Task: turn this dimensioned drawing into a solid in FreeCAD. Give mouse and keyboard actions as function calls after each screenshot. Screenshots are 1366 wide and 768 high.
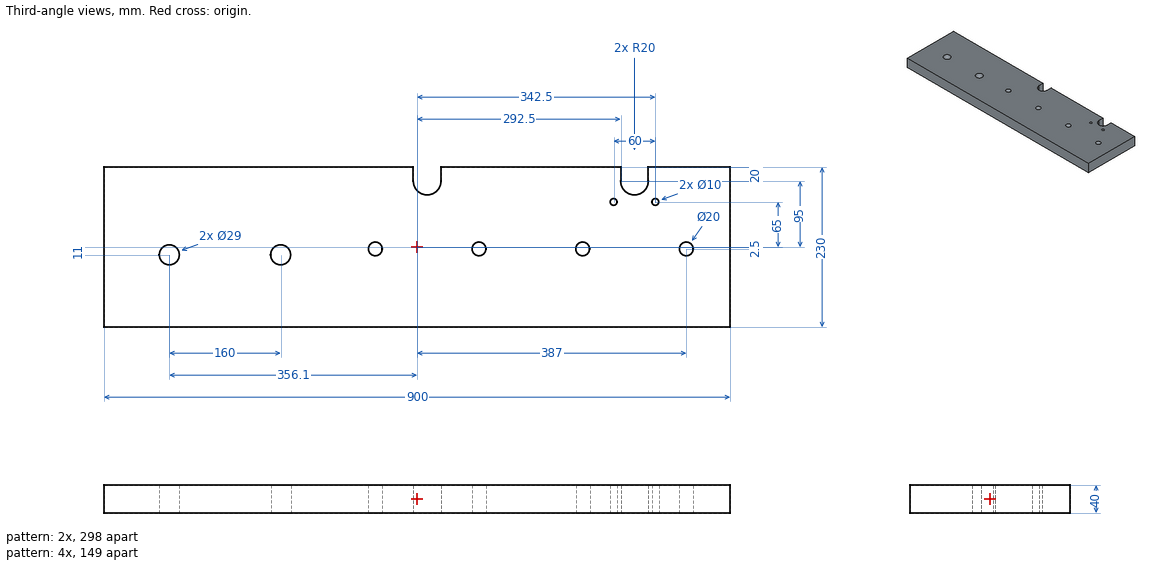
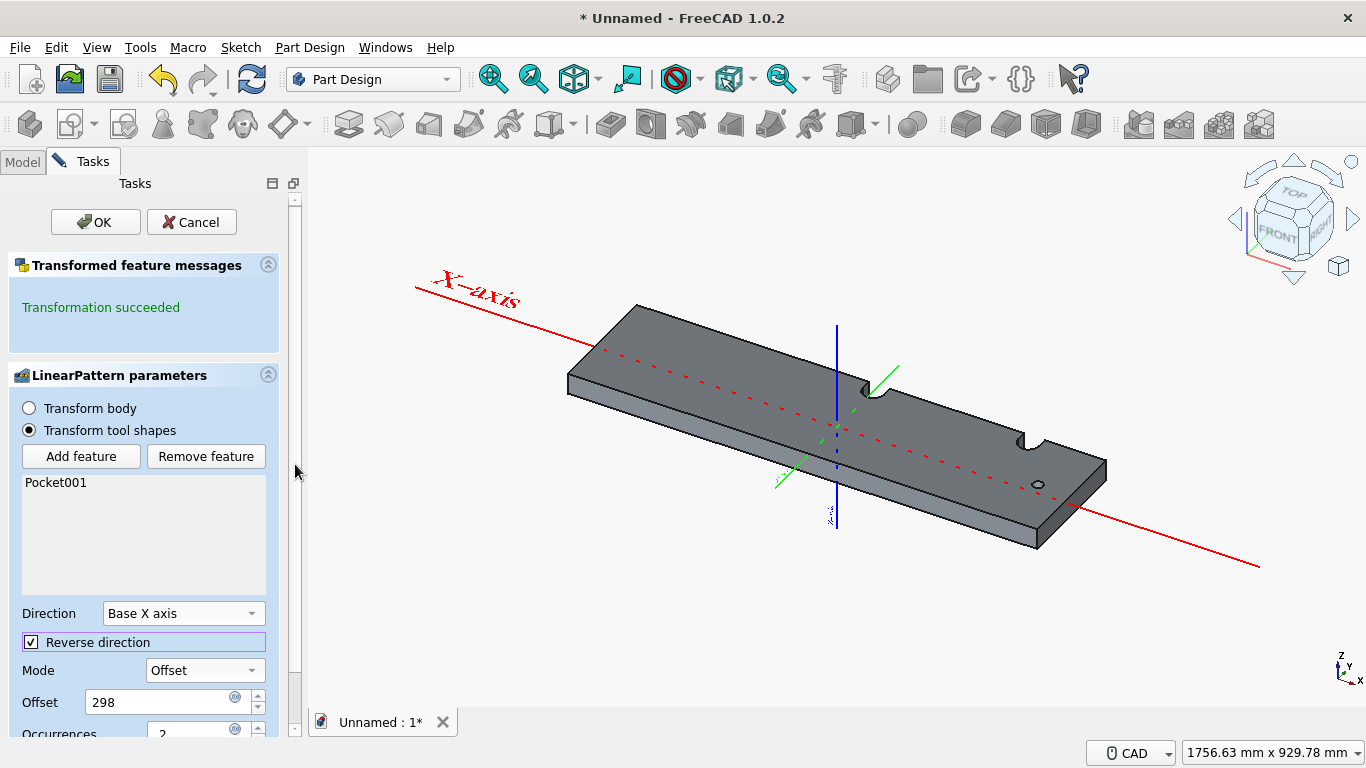
click(96, 222)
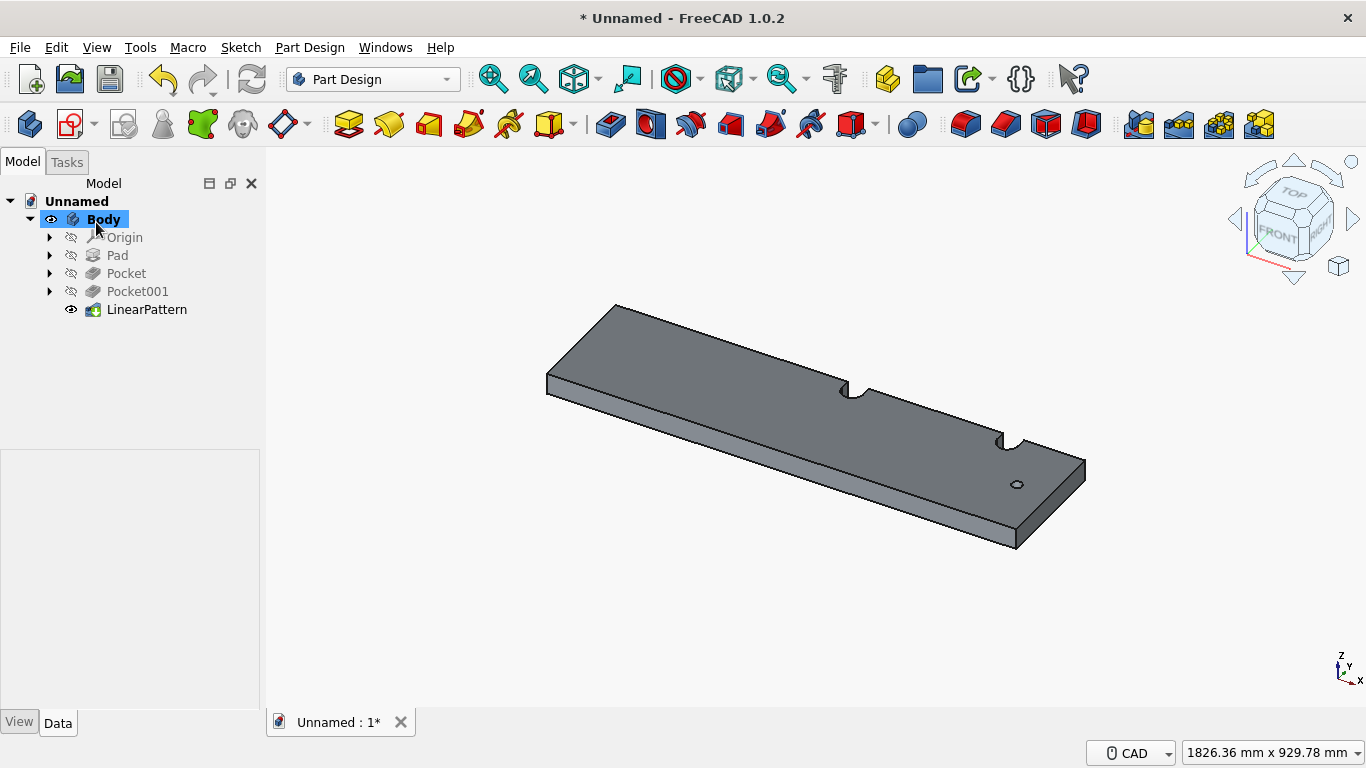
click(116, 273)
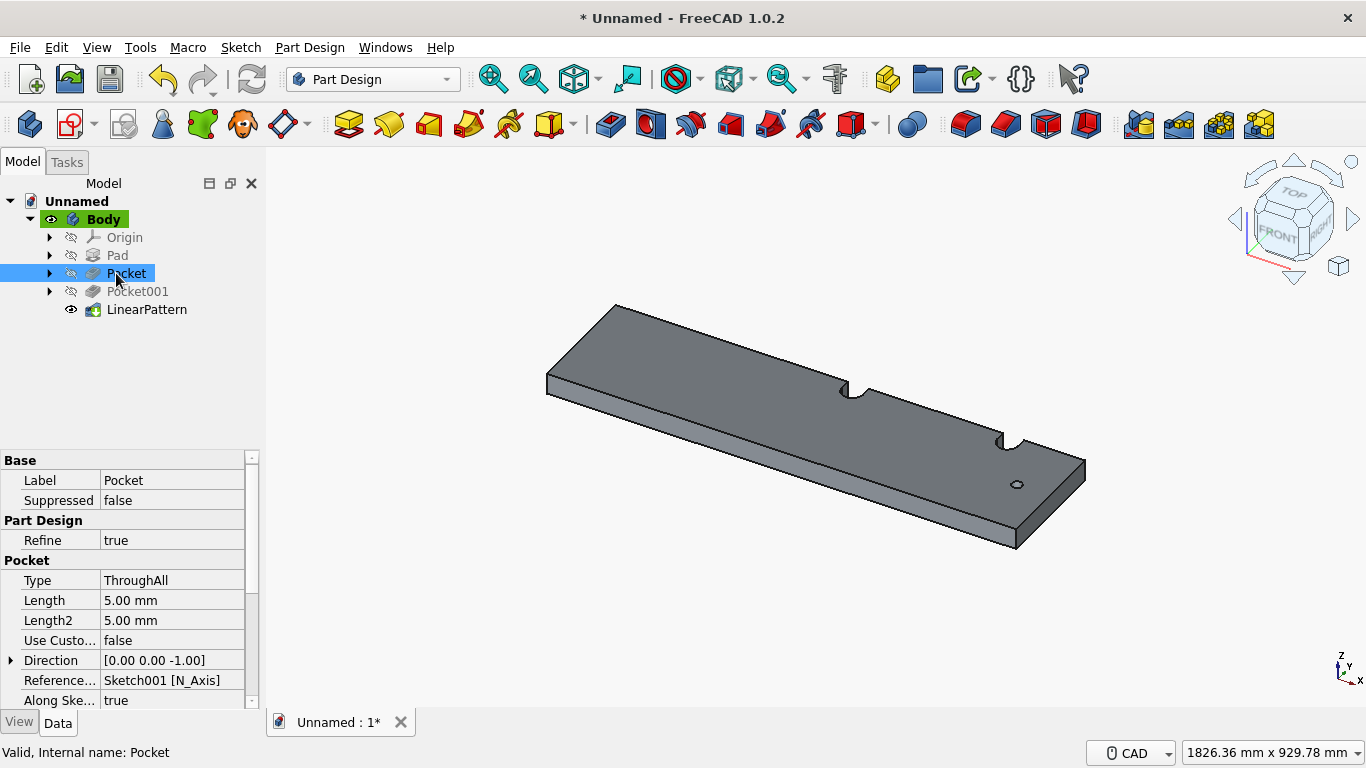
click(1180, 124)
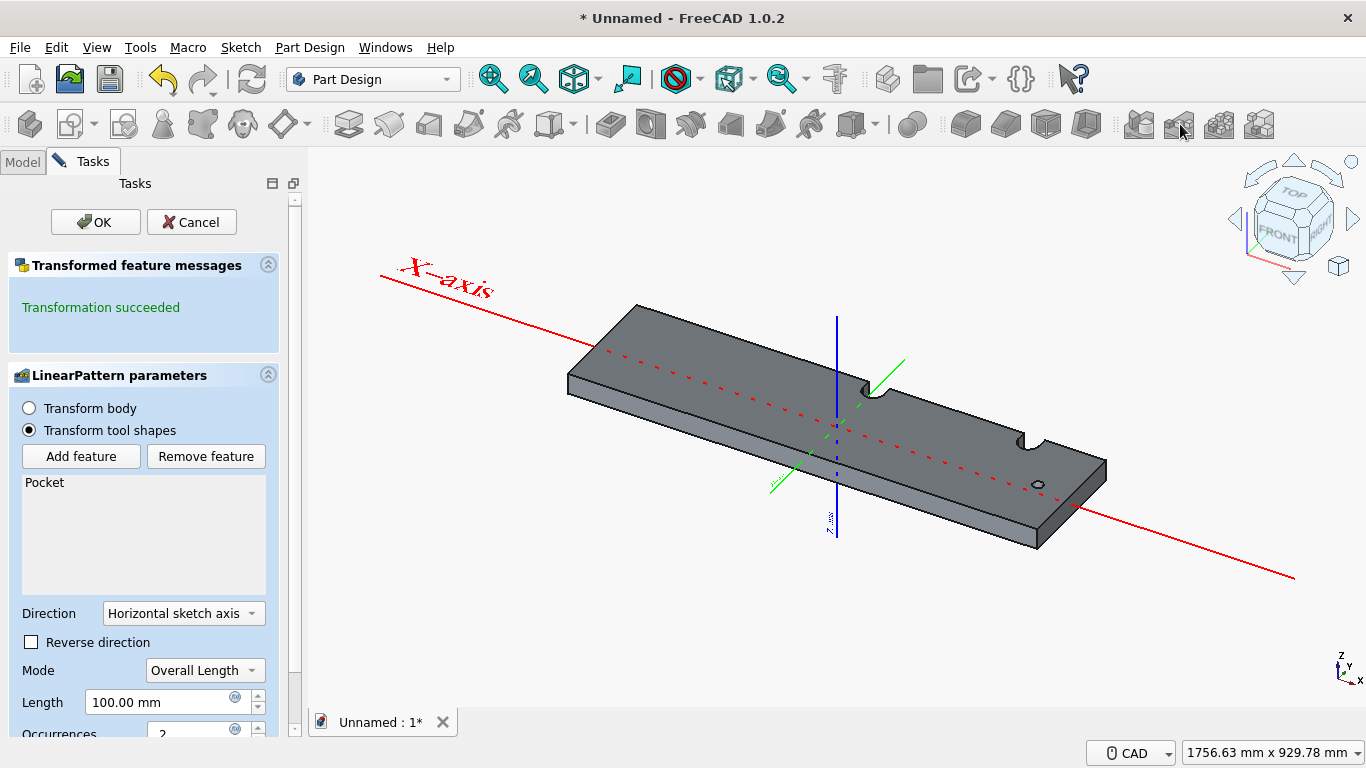
click(184, 614)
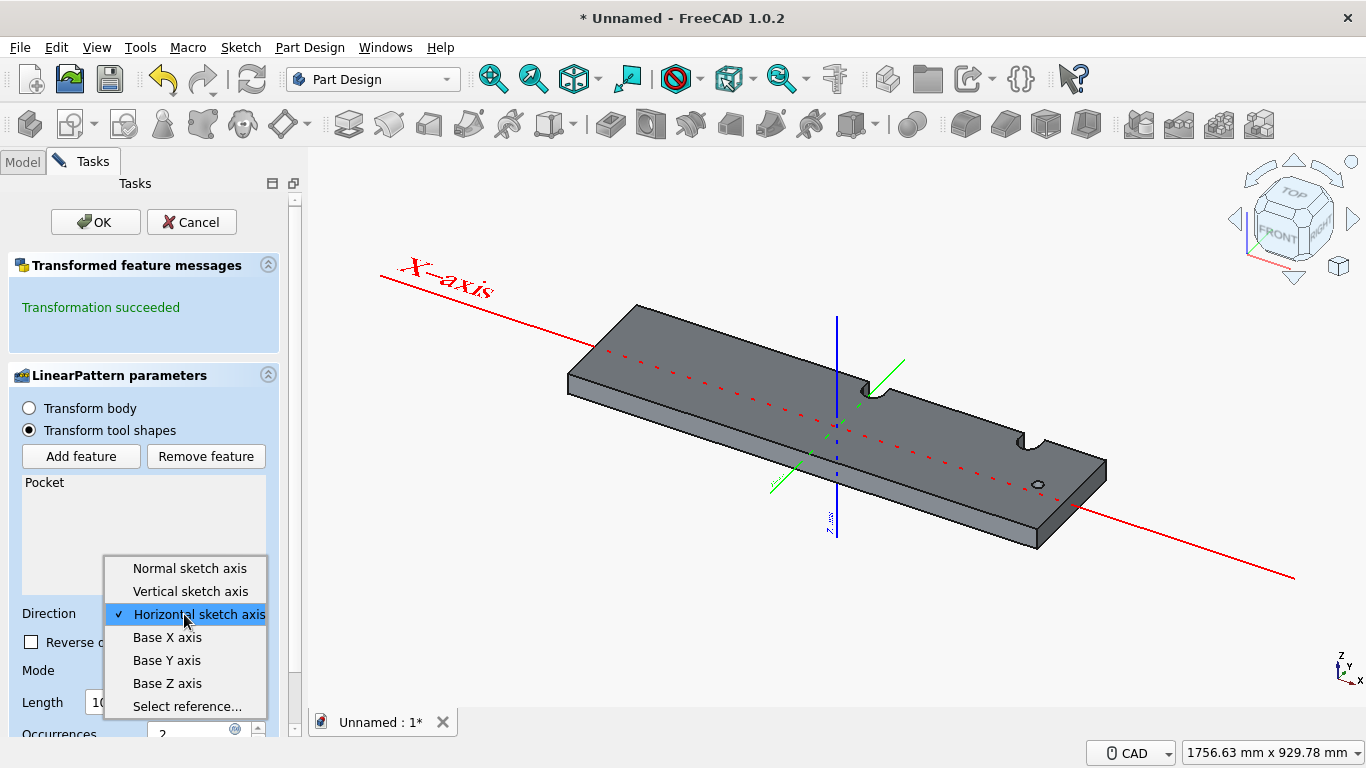
click(184, 638)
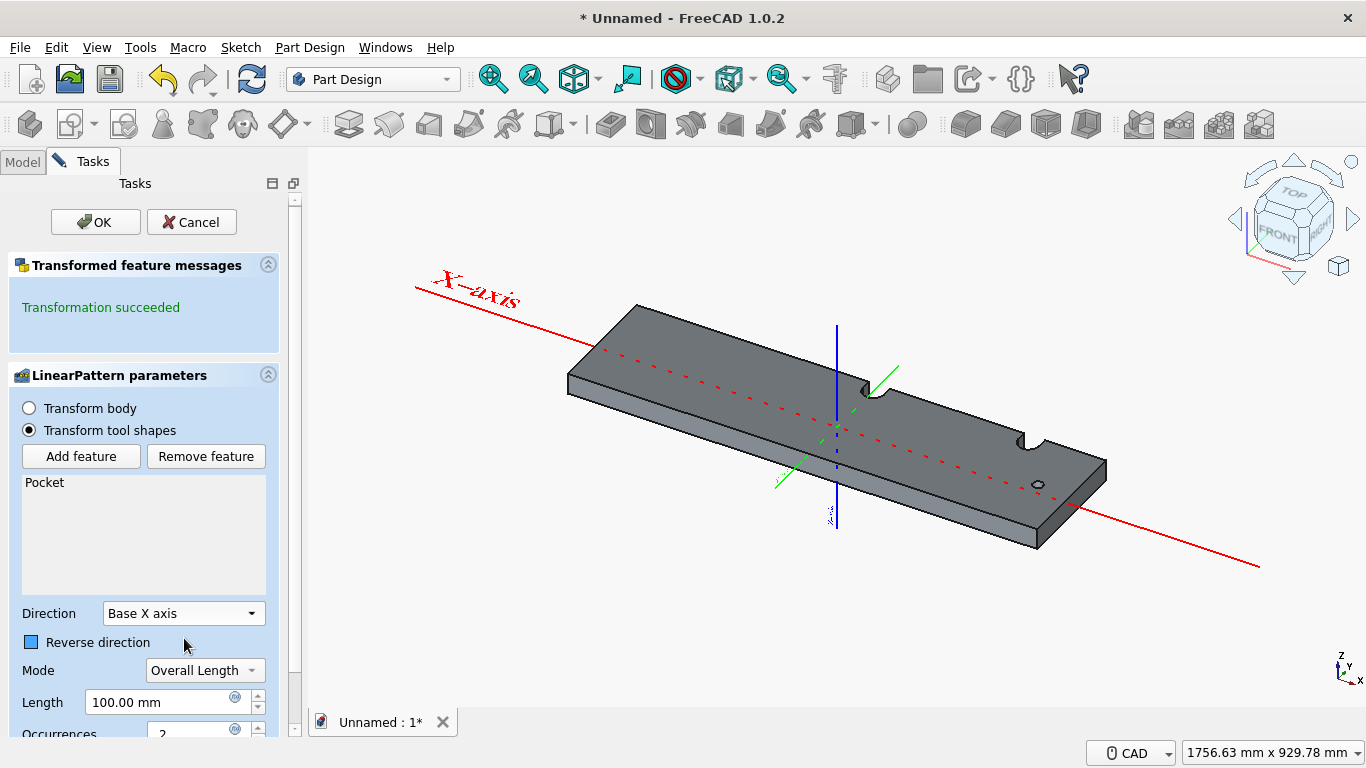
click(206, 670)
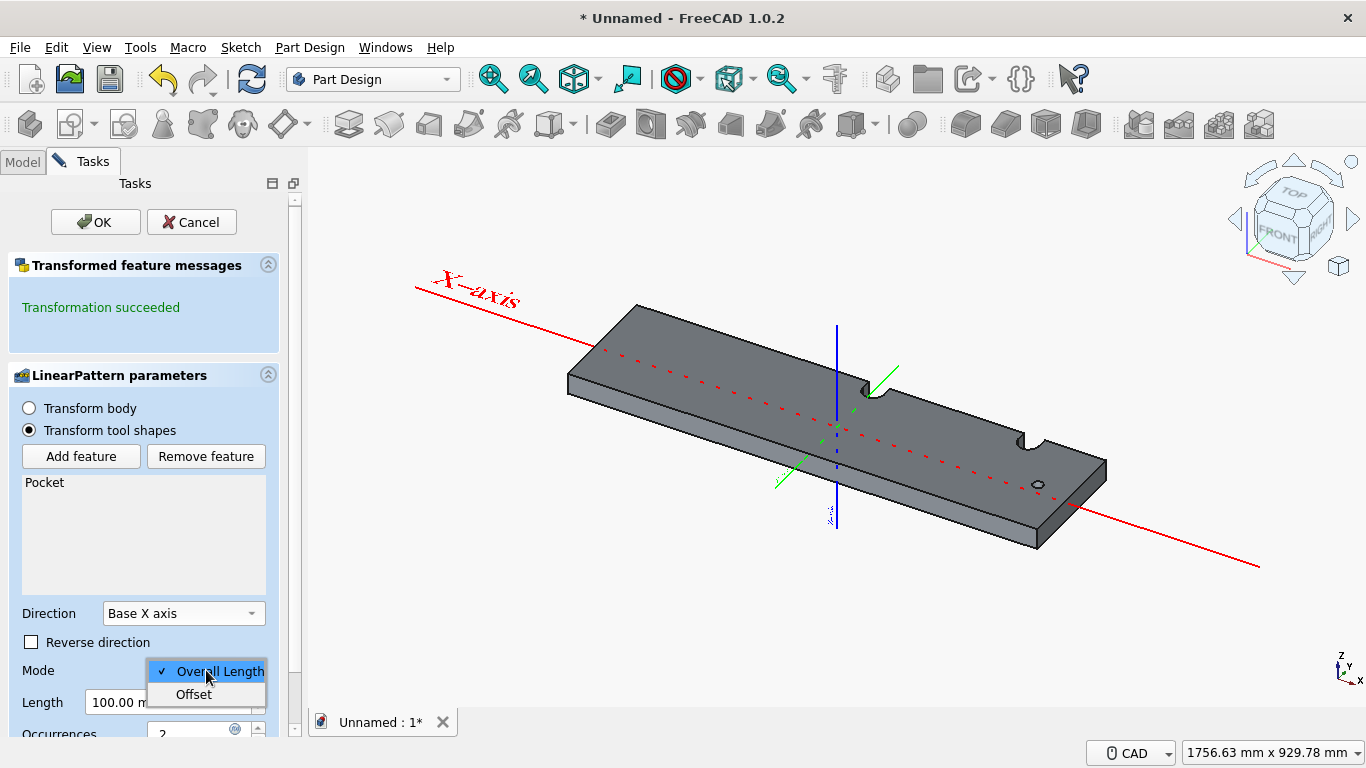
click(206, 694)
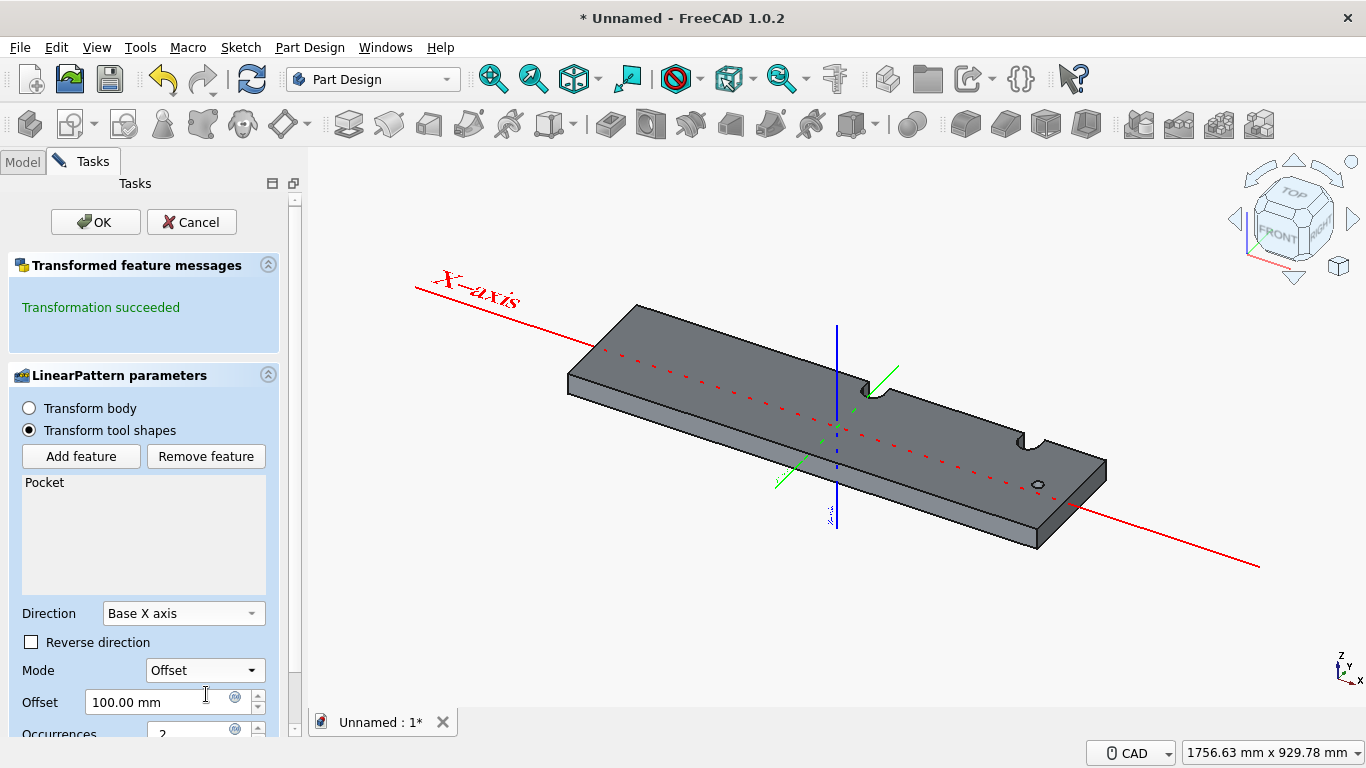
triple_click(168, 702)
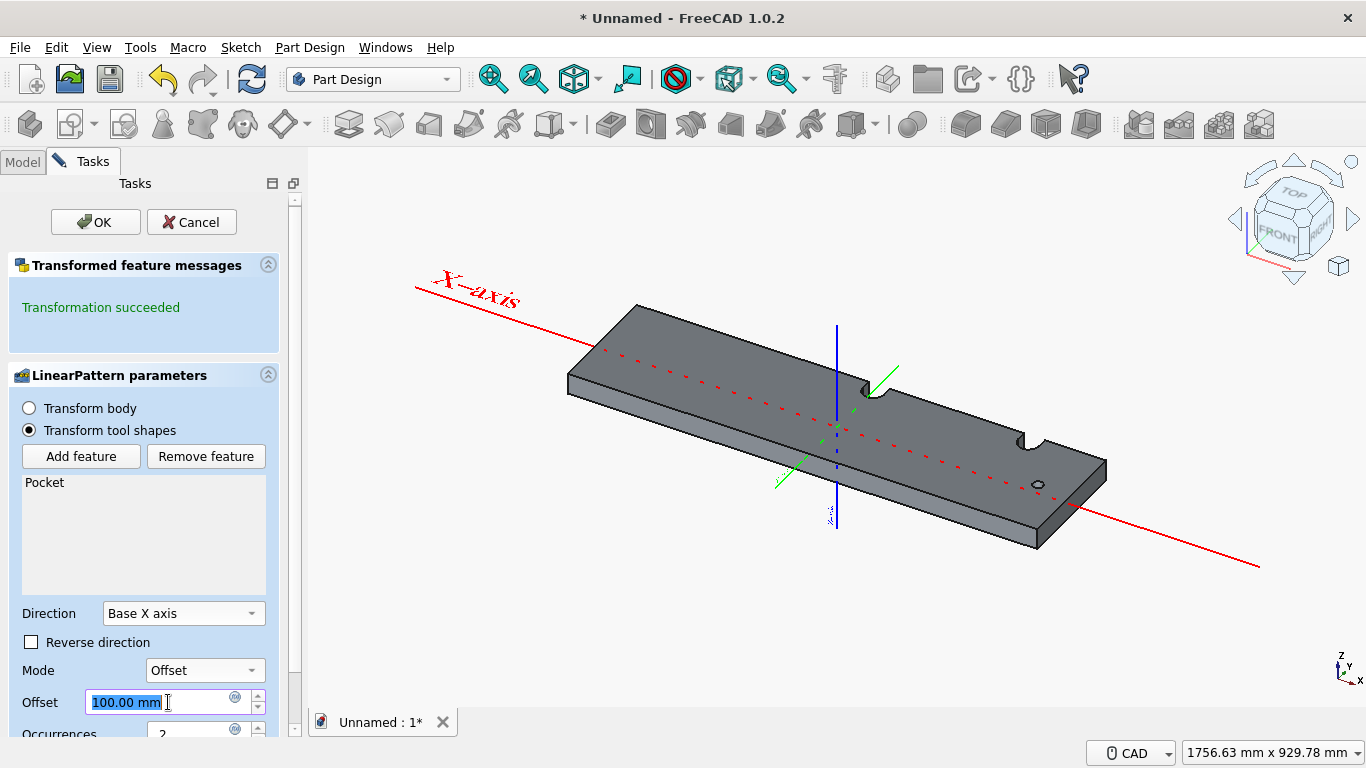
text(149)
key(Tab)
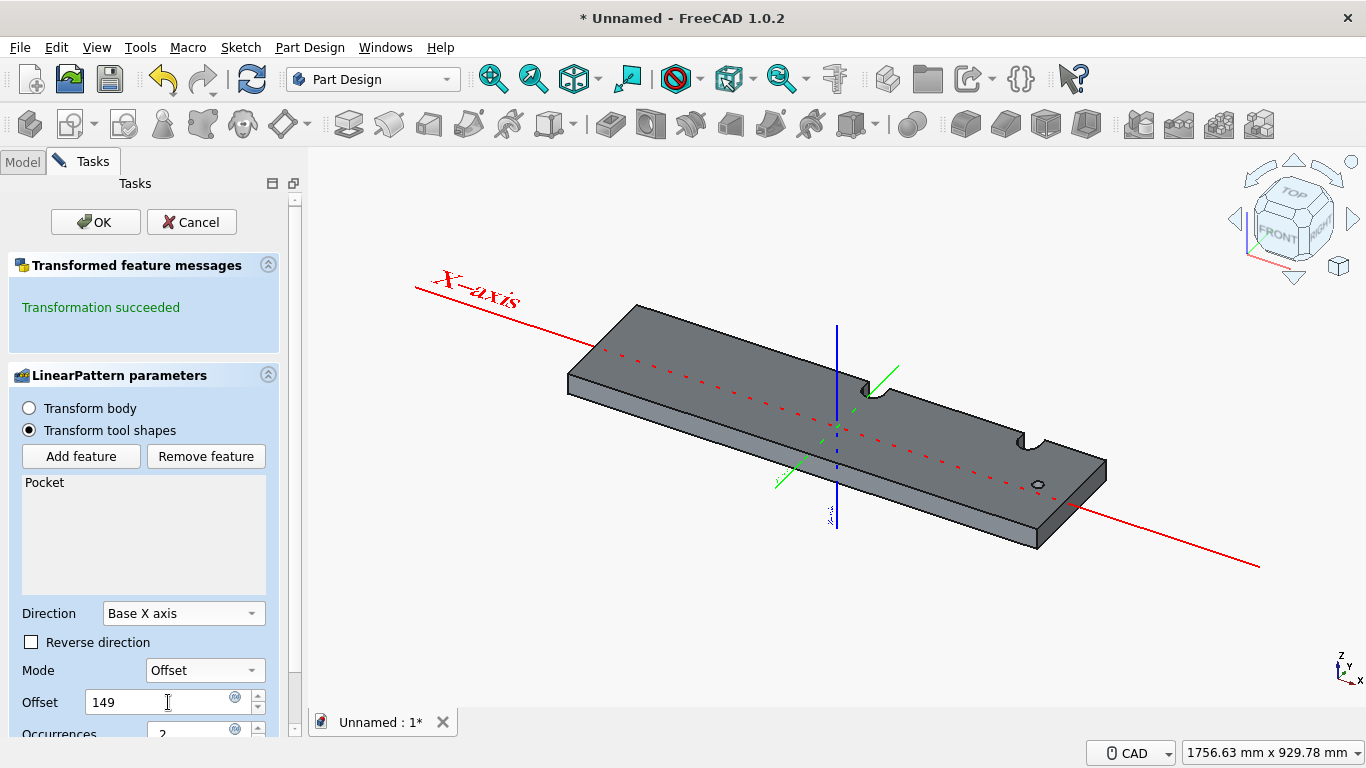
scroll(295, 464, down, 2)